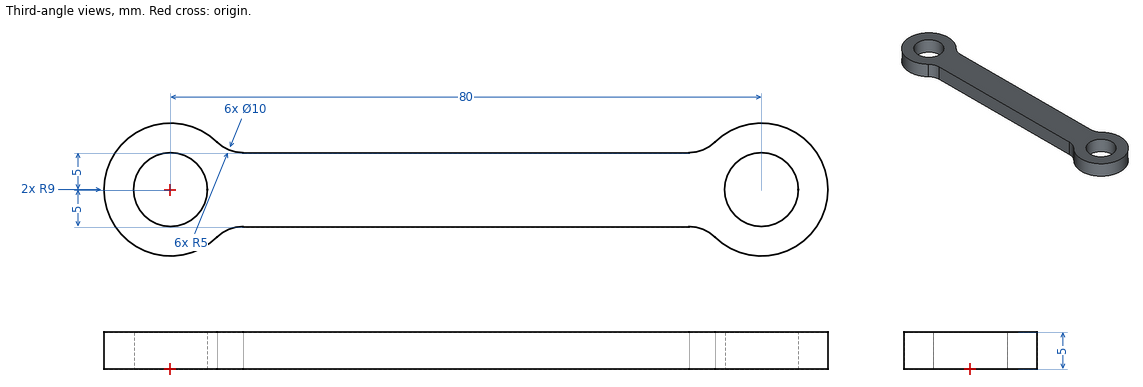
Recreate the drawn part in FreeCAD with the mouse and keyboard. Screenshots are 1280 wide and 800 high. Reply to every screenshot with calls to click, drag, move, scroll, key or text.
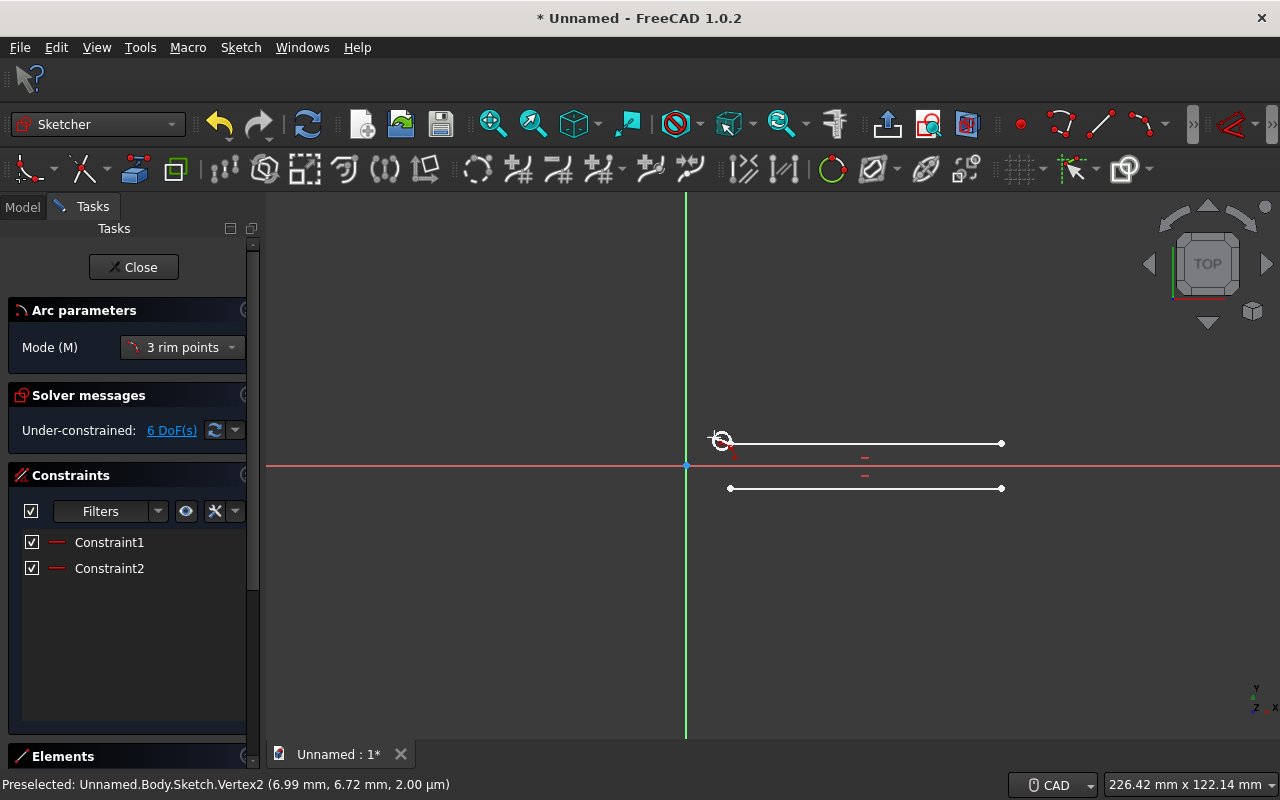
scroll(722, 441, up, 12)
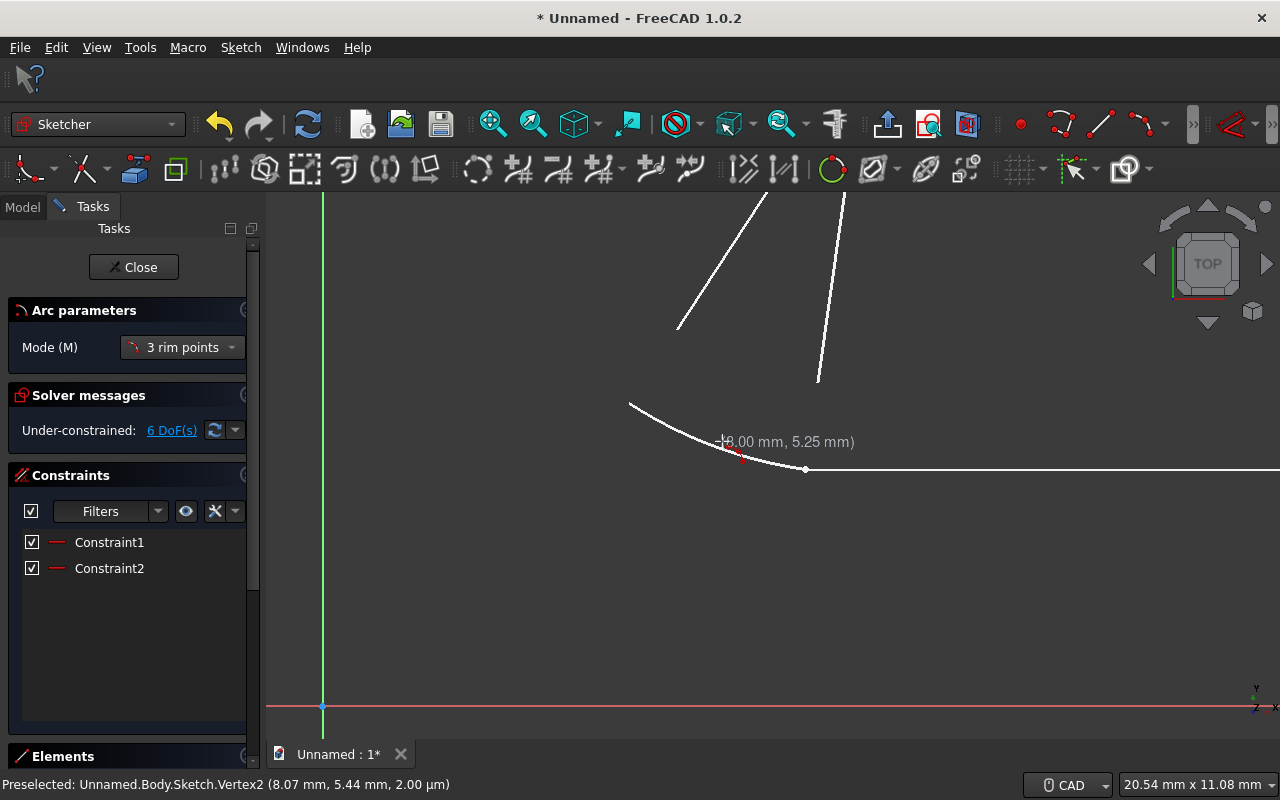
click(713, 441)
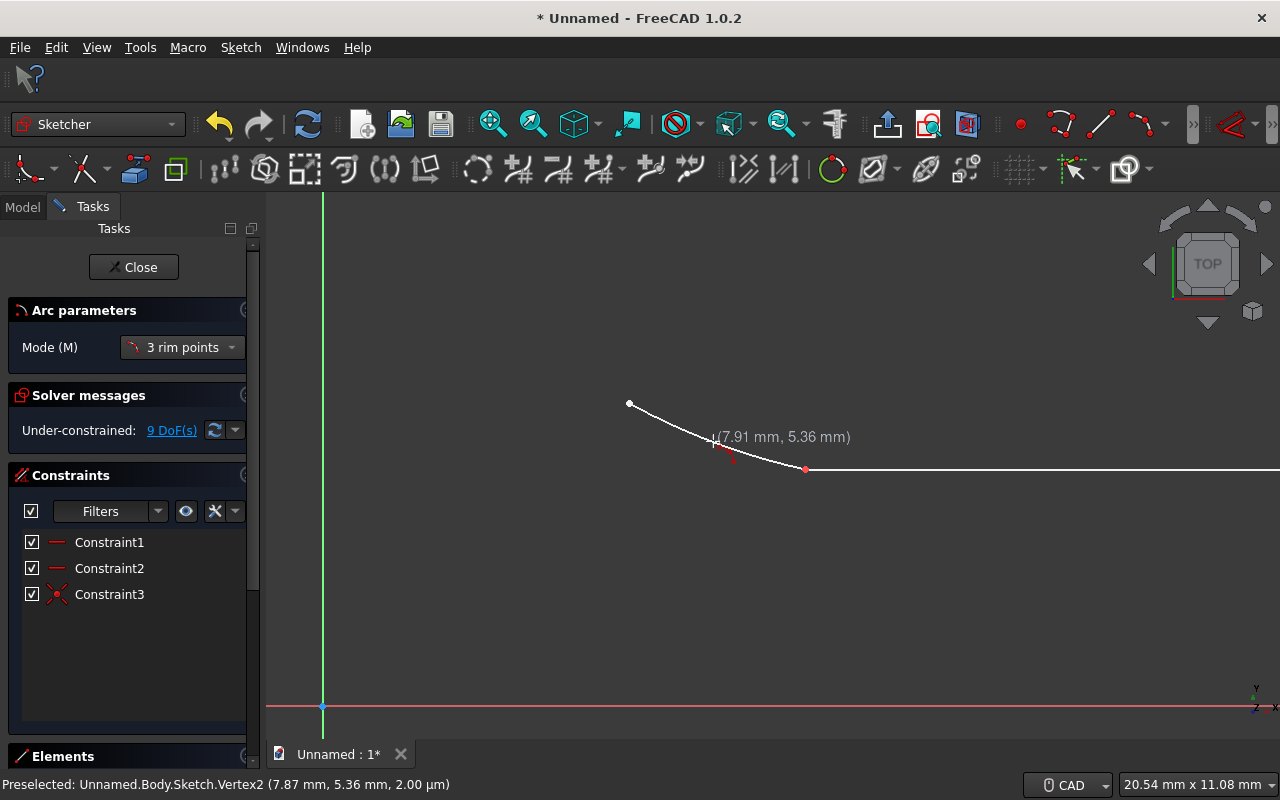
scroll(506, 435, down, 11)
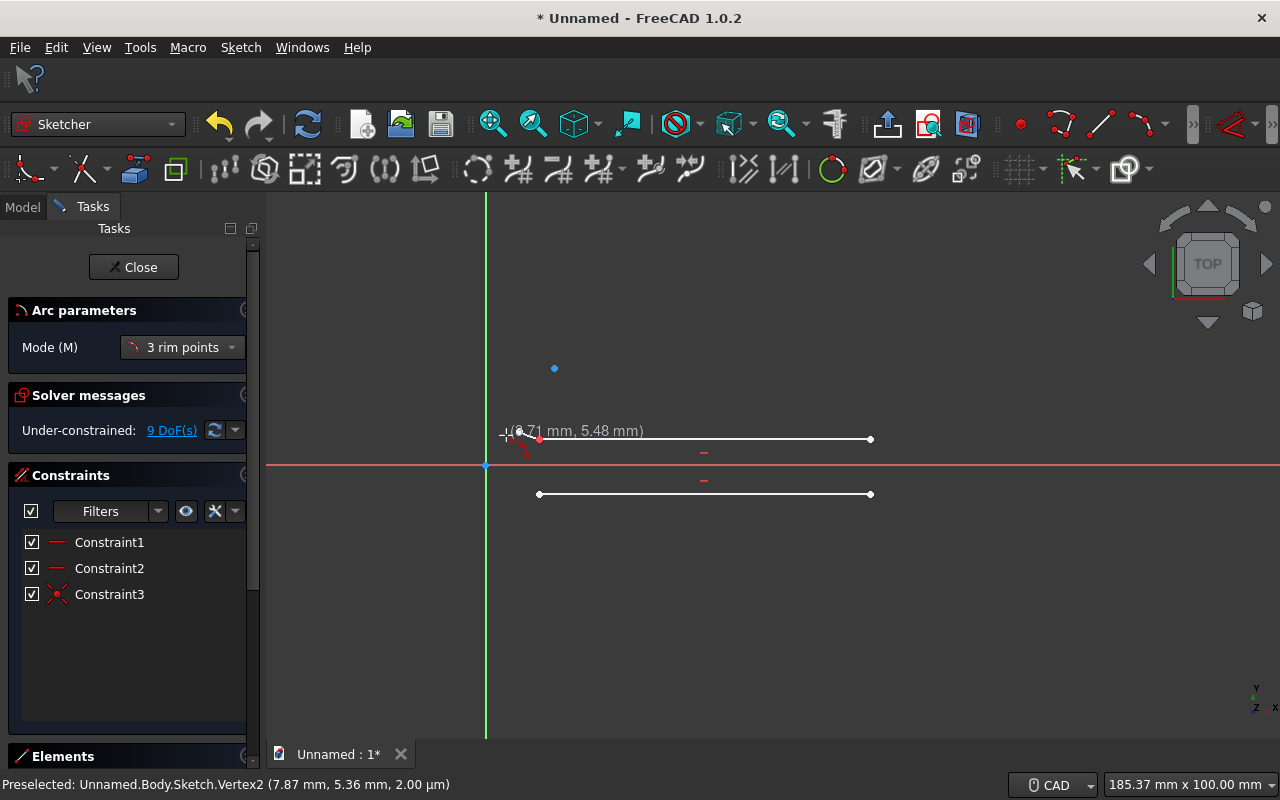
click(520, 432)
click(520, 501)
click(442, 443)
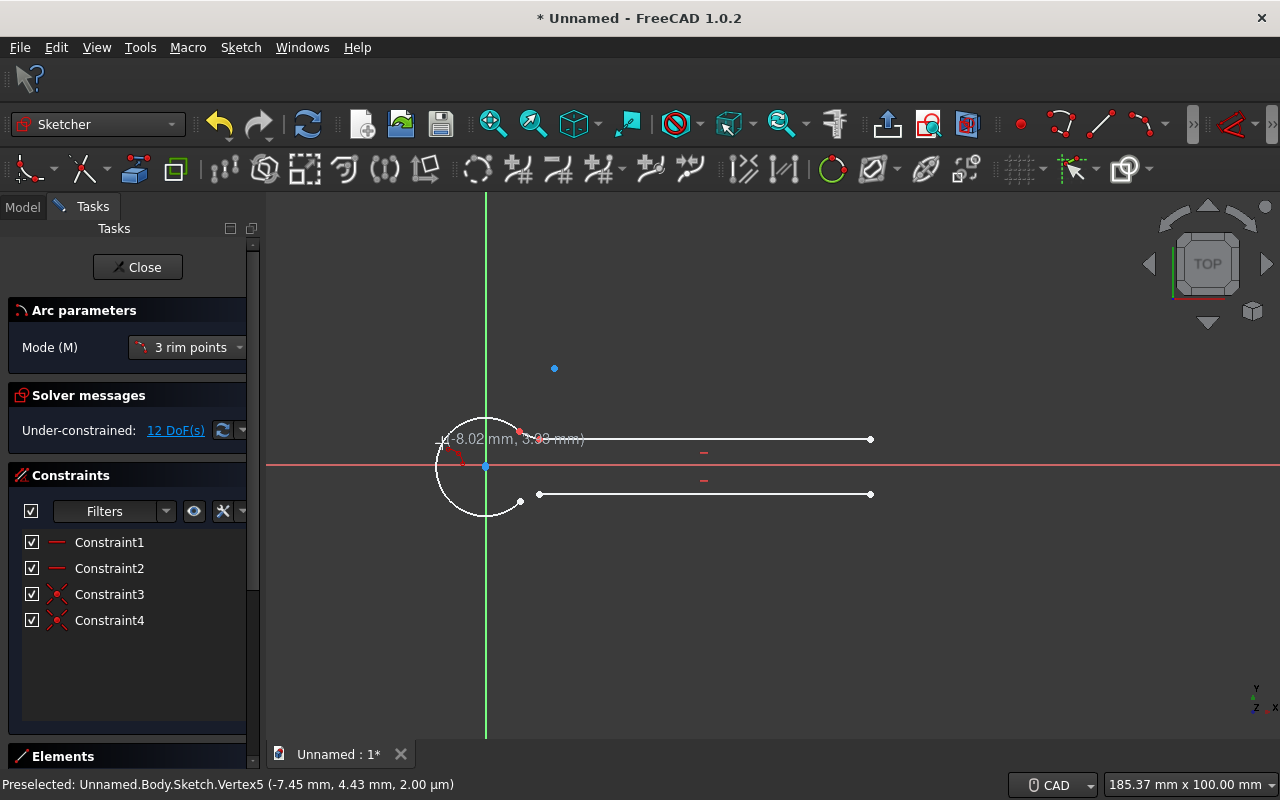
click(520, 502)
click(539, 494)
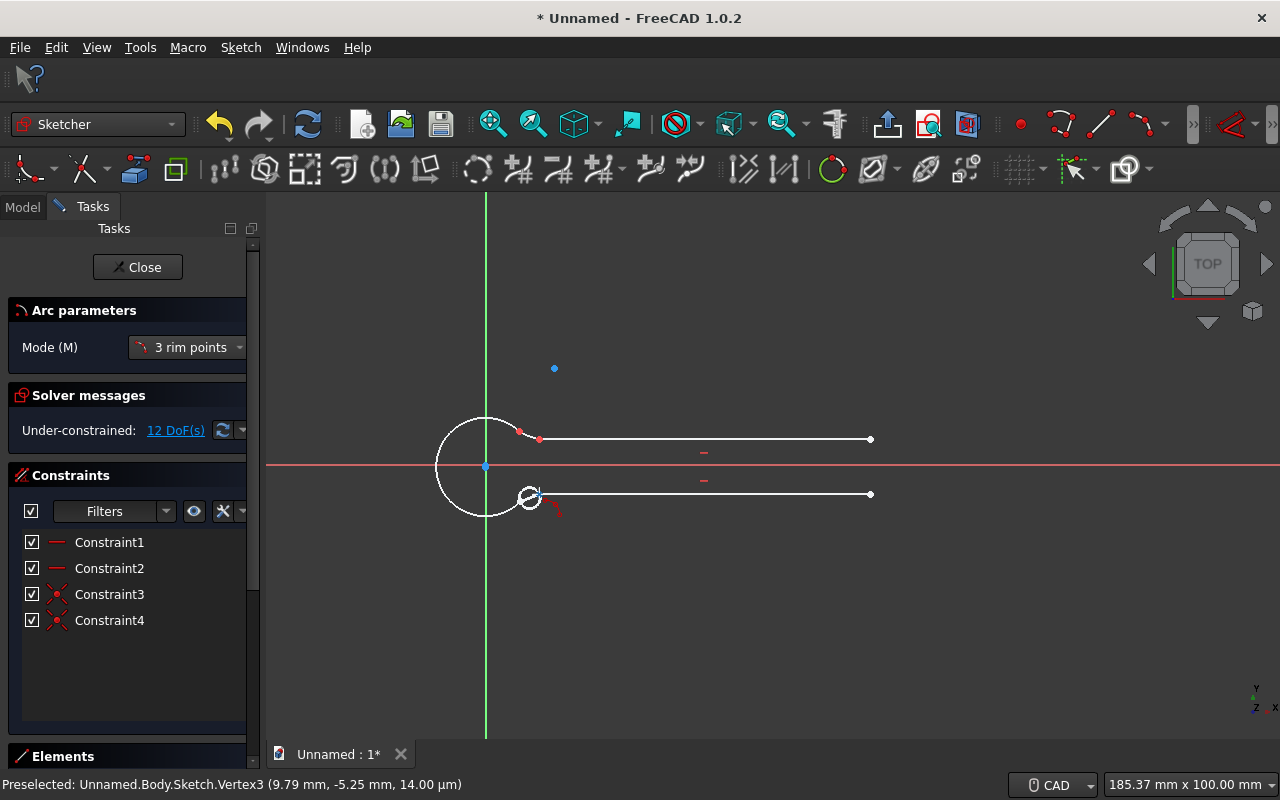
scroll(529, 495, up, 11)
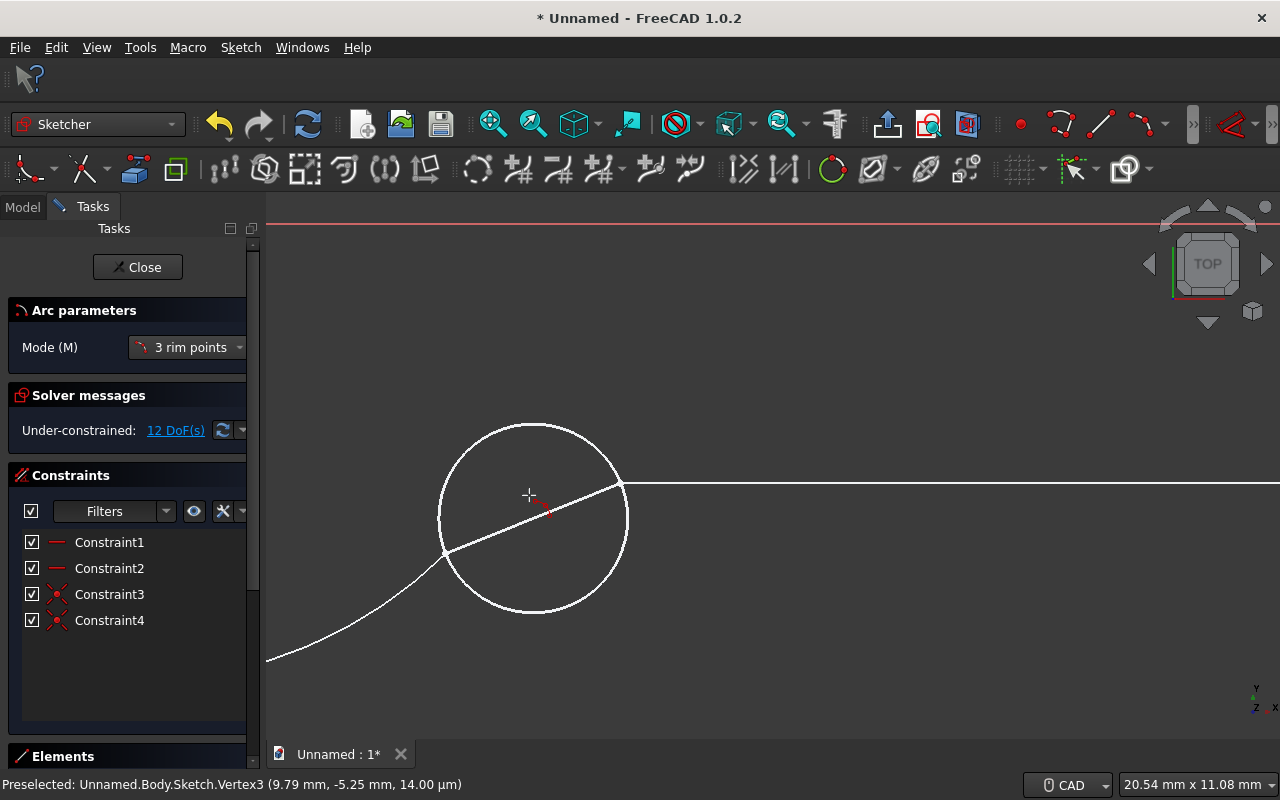
click(528, 489)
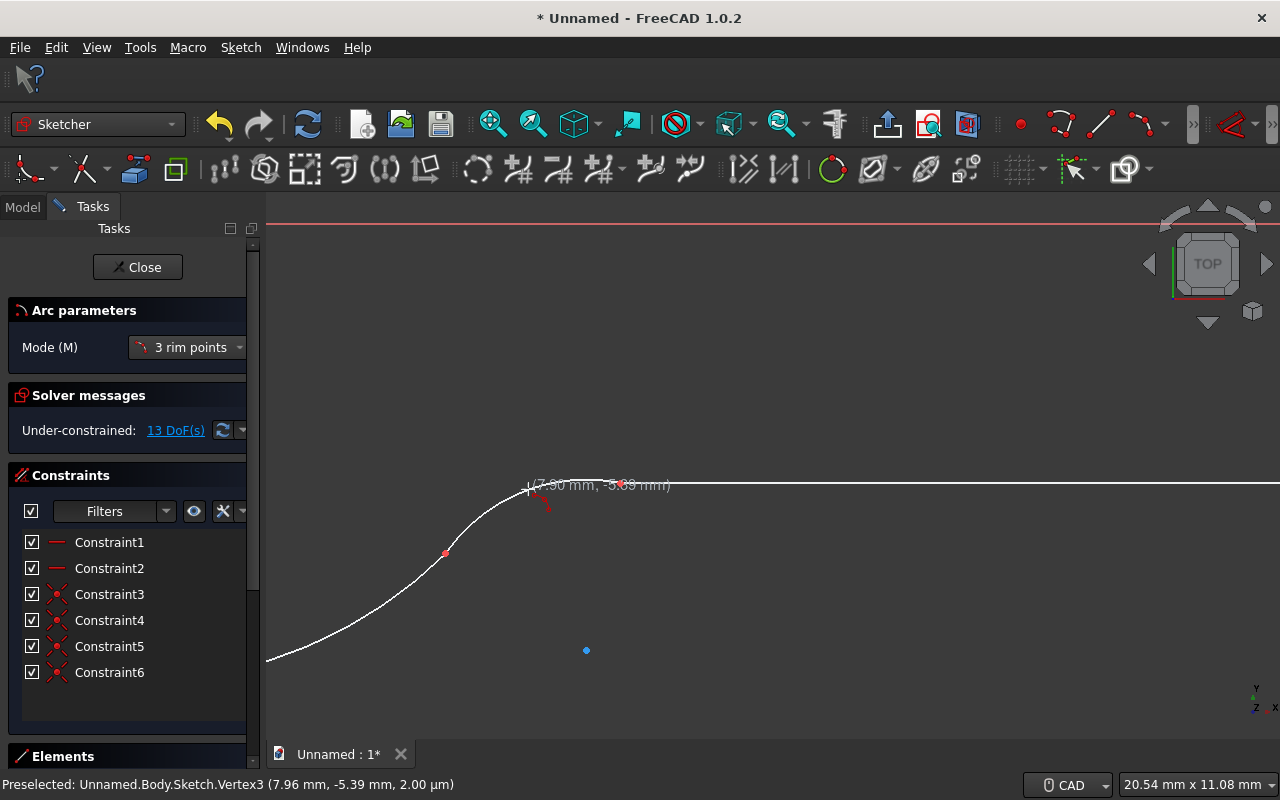
scroll(529, 496, down, 11)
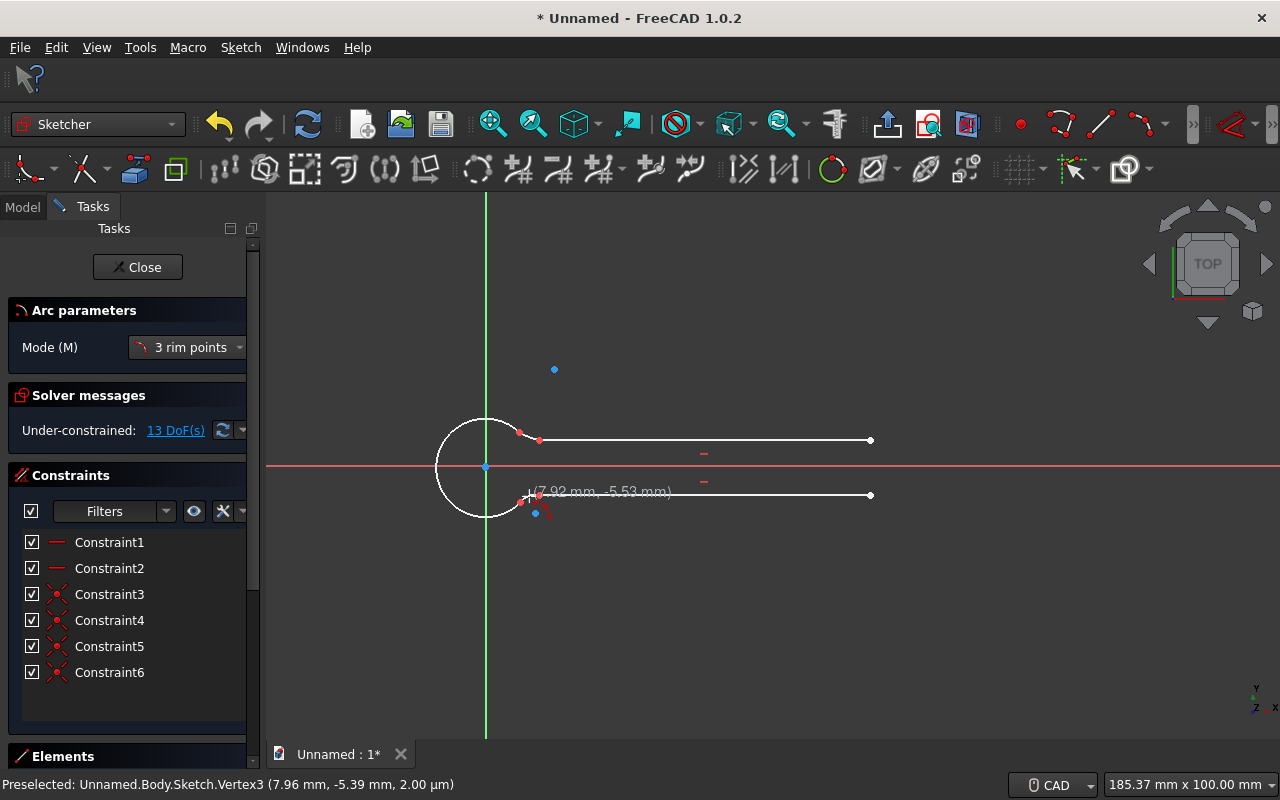
click(870, 495)
click(889, 502)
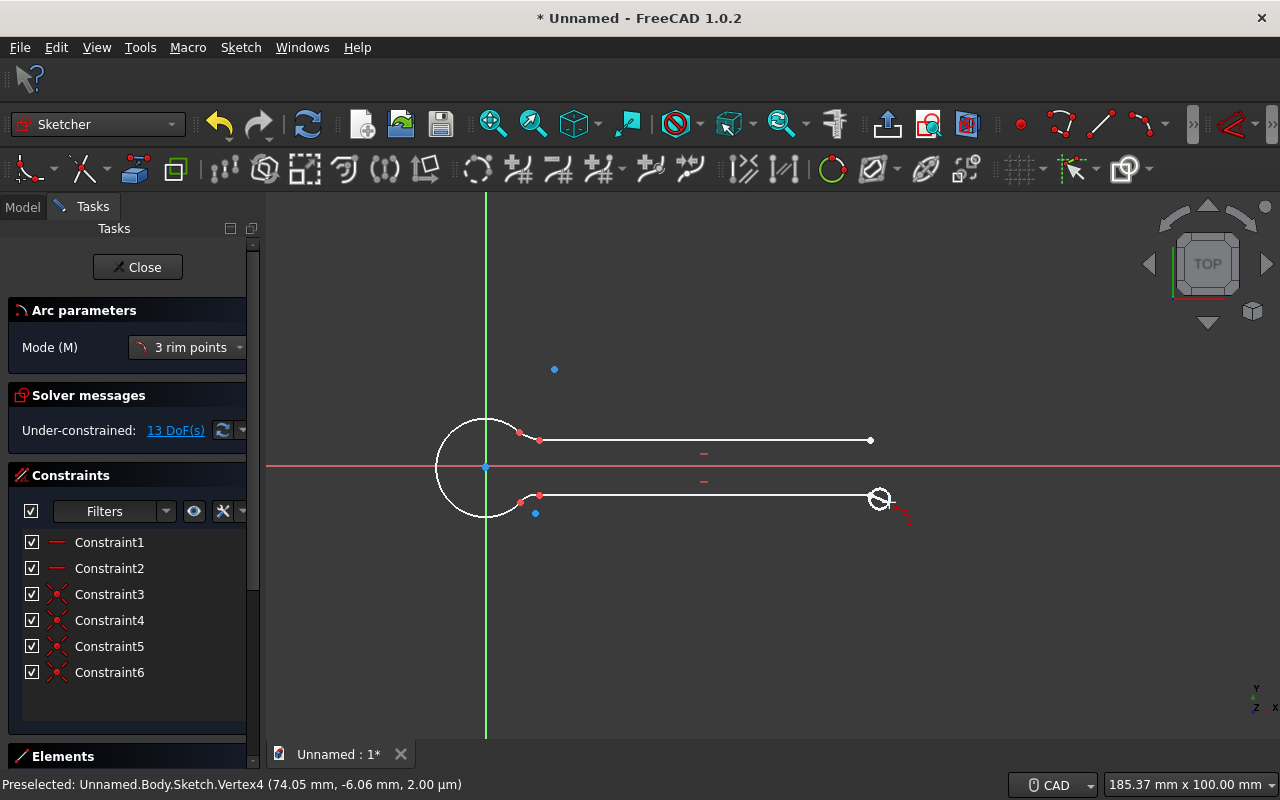
scroll(880, 496, up, 11)